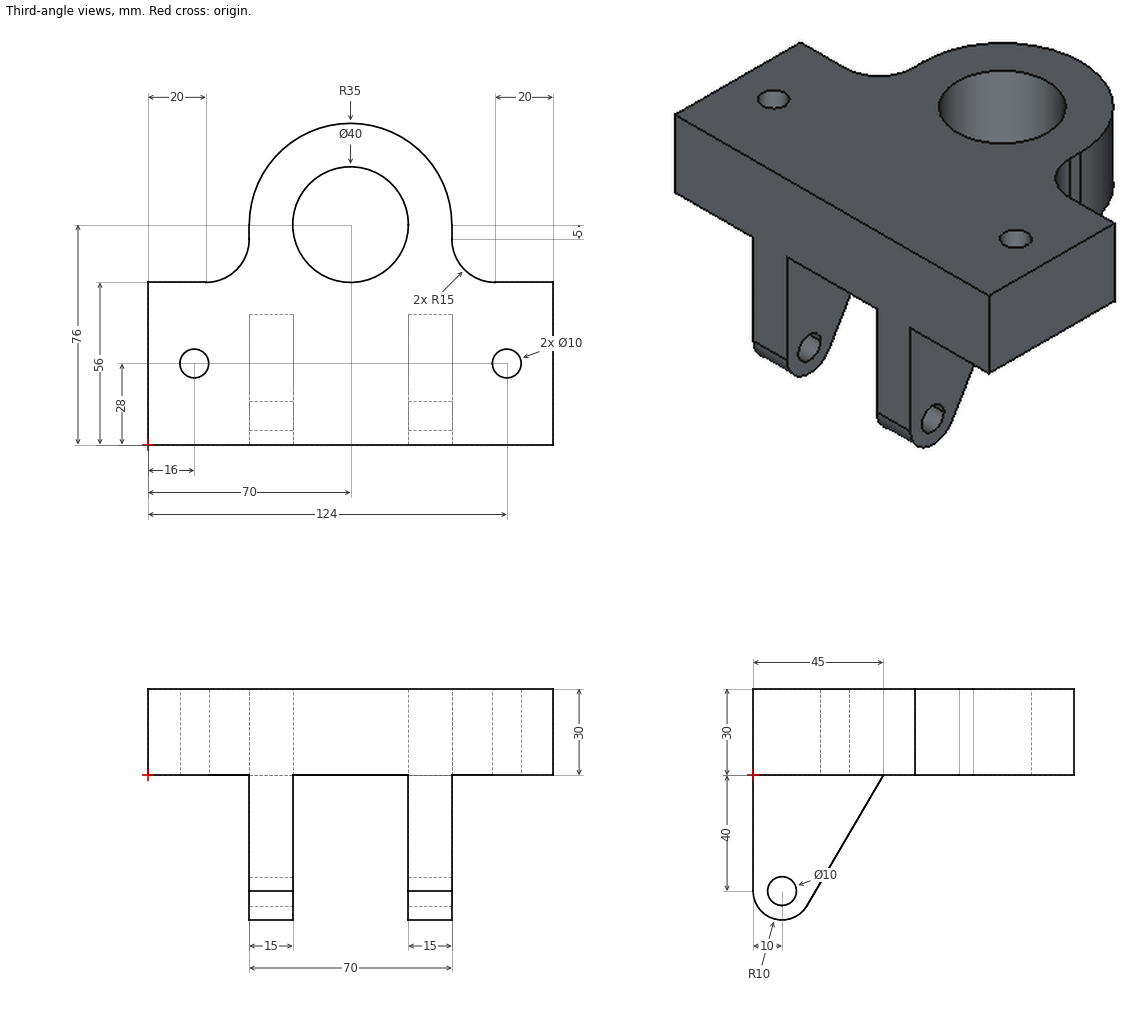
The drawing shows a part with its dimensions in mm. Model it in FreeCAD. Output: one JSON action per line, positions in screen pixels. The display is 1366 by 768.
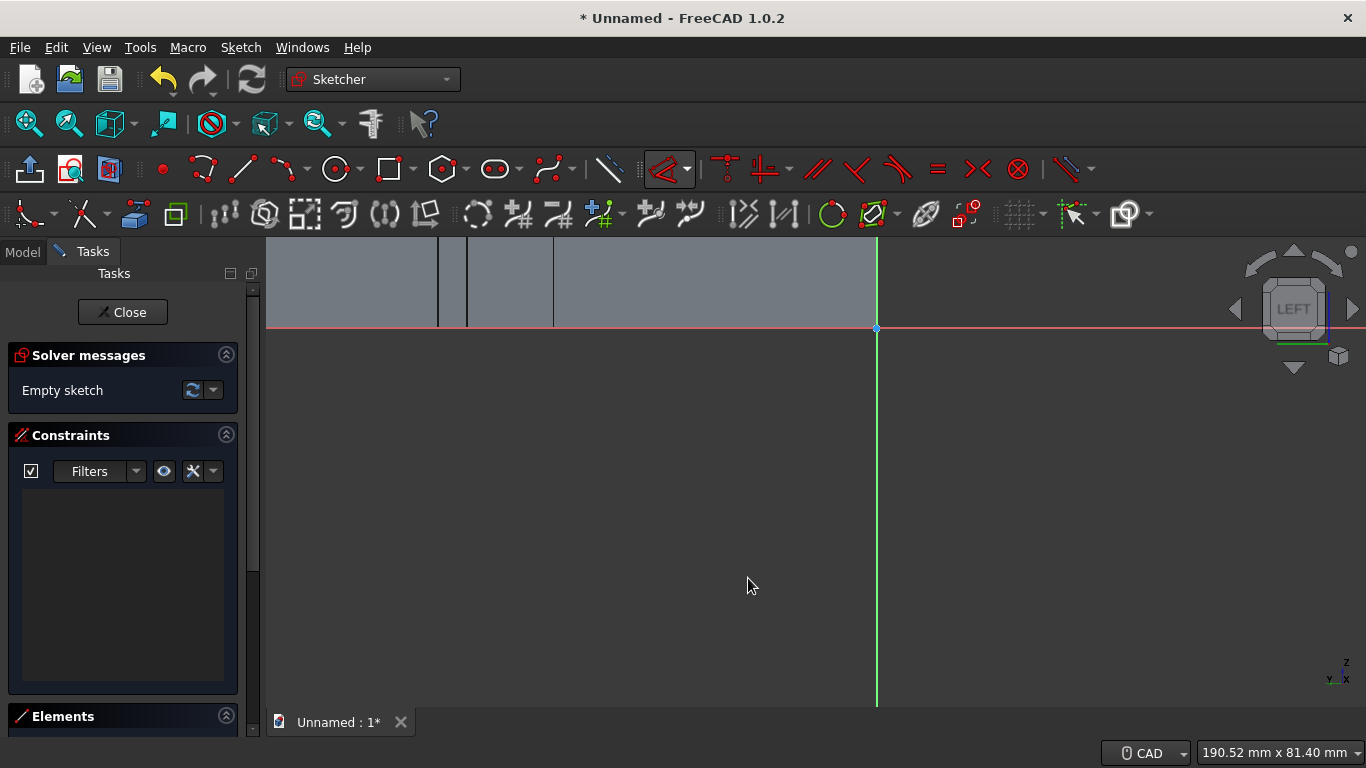
{"action": "left_click", "coordinate": [204, 170]}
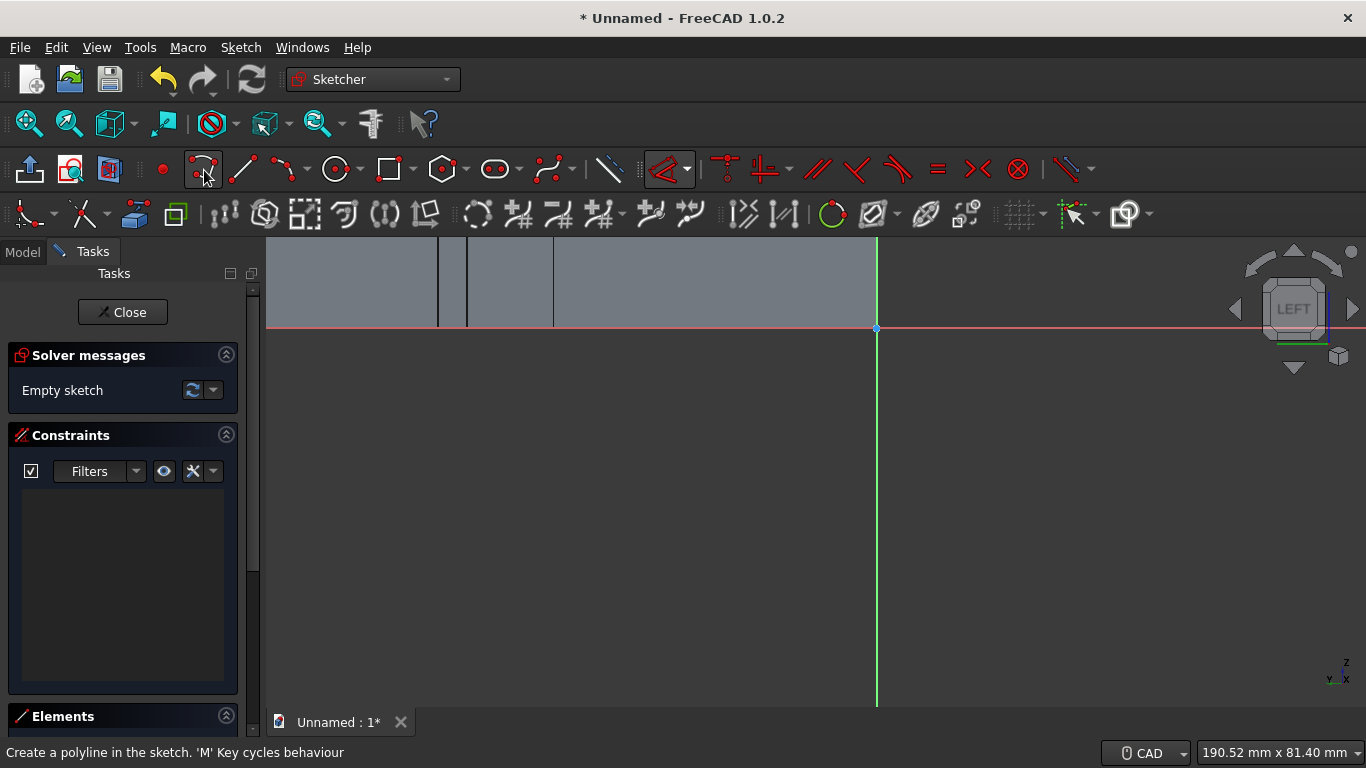
{"action": "left_click", "coordinate": [769, 588]}
{"action": "left_click", "coordinate": [617, 328]}
{"action": "left_click", "coordinate": [877, 328]}
{"action": "left_click", "coordinate": [868, 559]}
{"action": "right_click", "coordinate": [868, 559]}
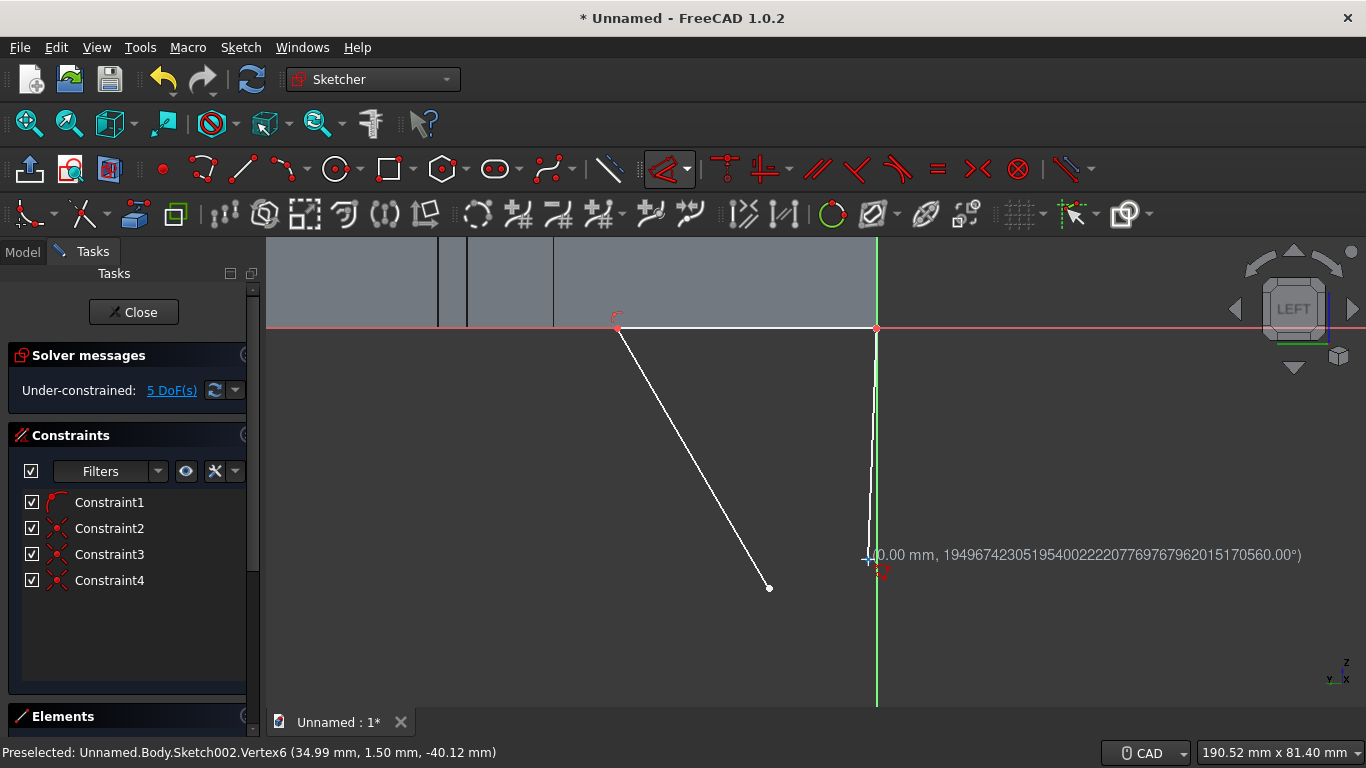
{"action": "key", "text": "g 3 a"}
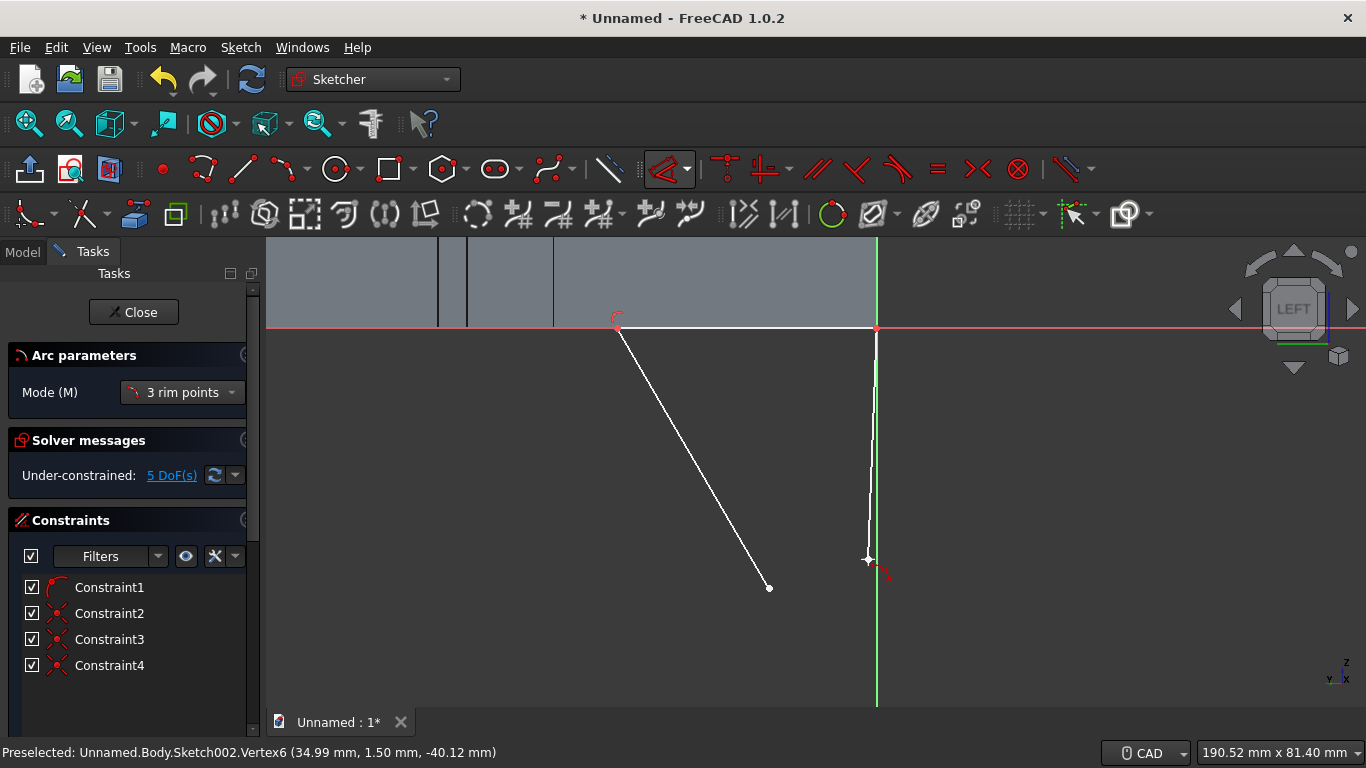
{"action": "left_click", "coordinate": [868, 560]}
{"action": "left_click", "coordinate": [769, 589]}
{"action": "left_click", "coordinate": [834, 615]}
{"action": "key", "text": "Escape"}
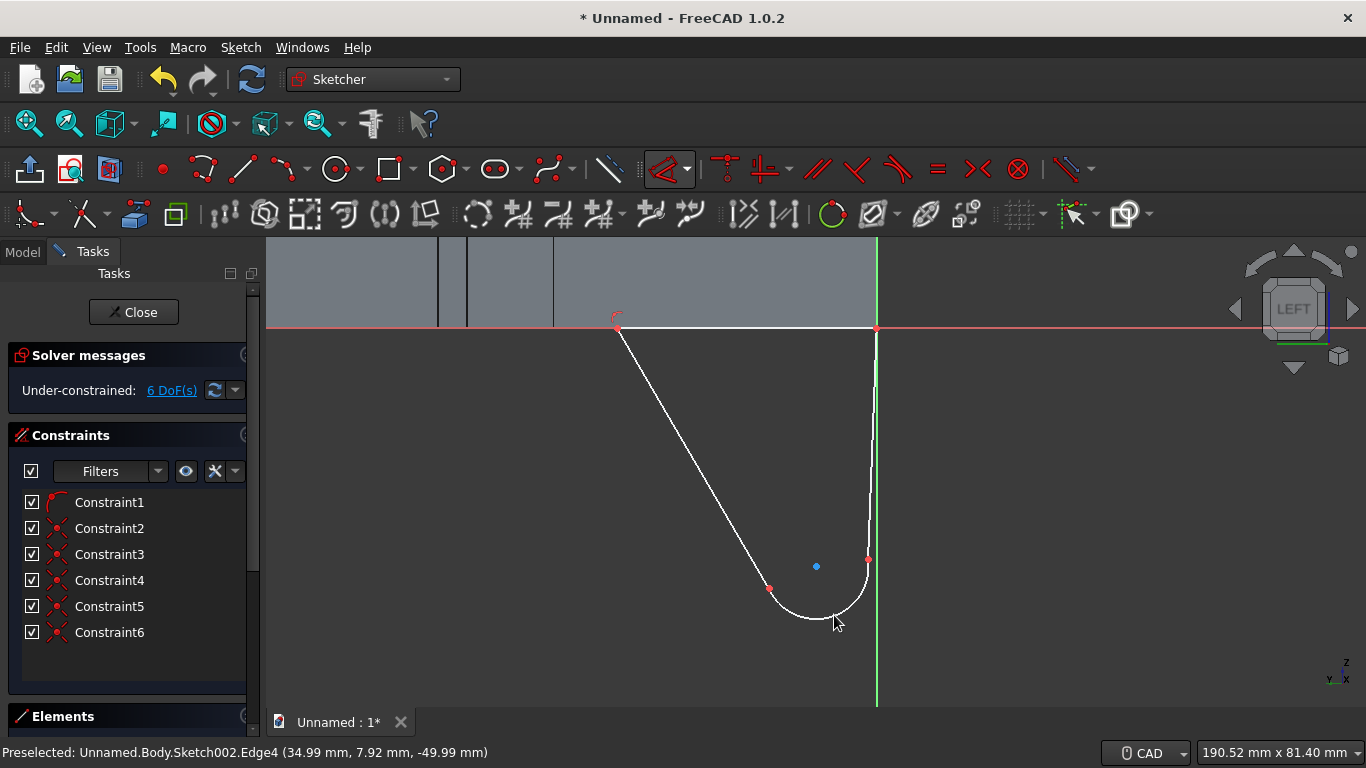
{"action": "left_click", "coordinate": [723, 511]}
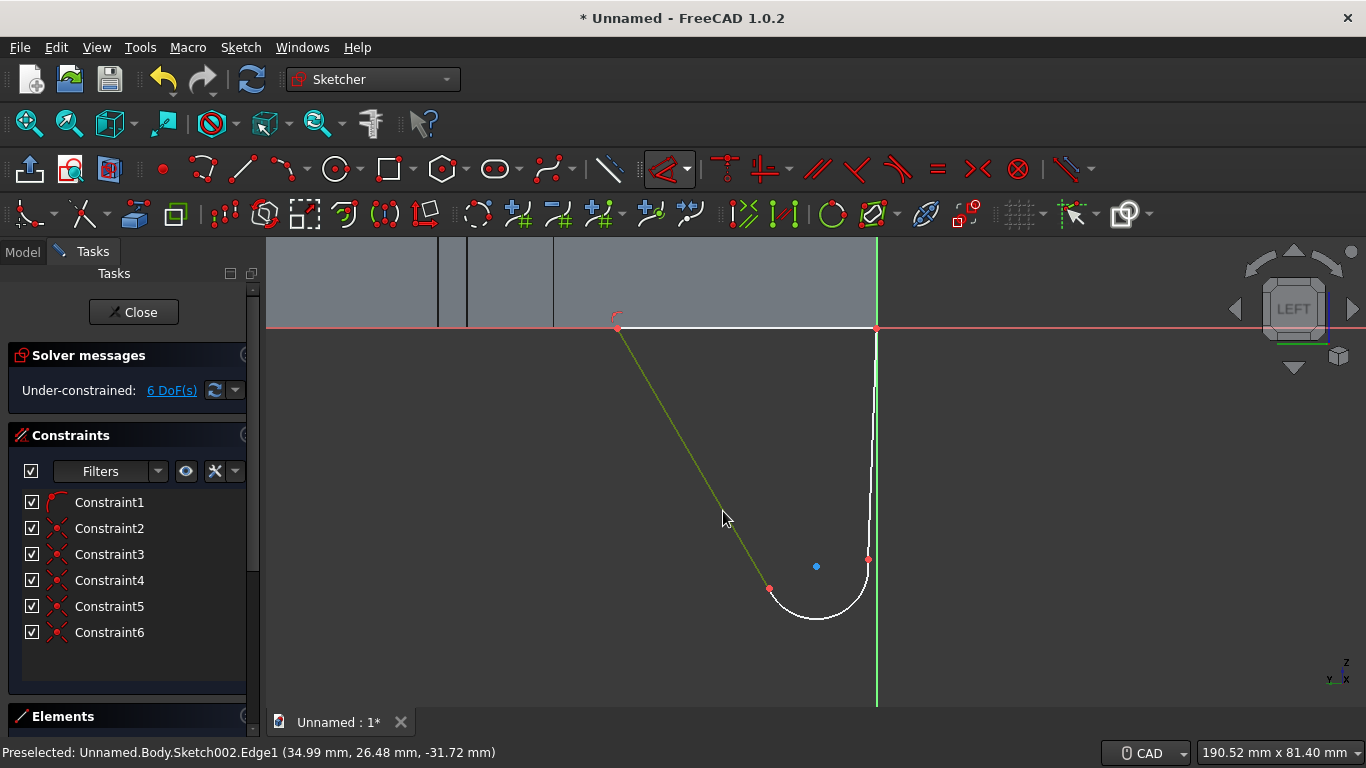
{"action": "left_click", "coordinate": [802, 617]}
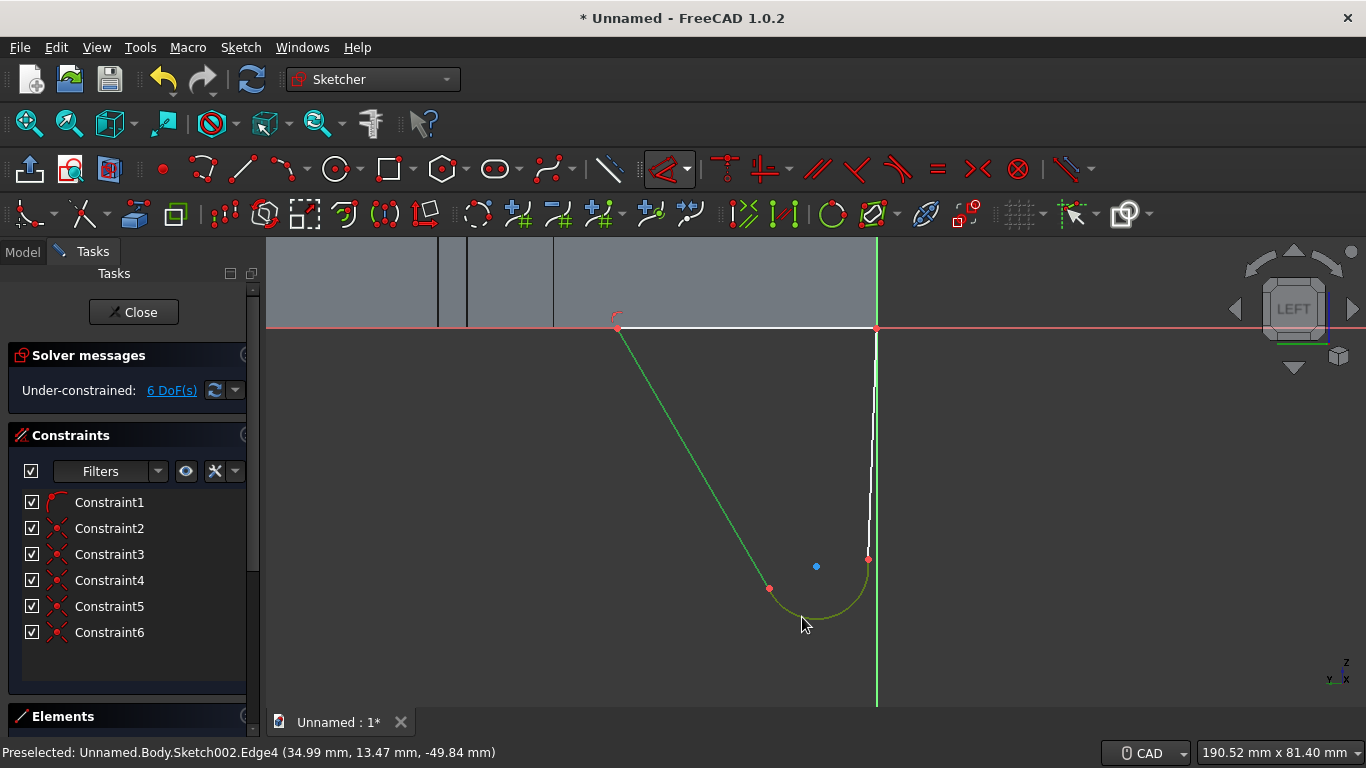
{"action": "left_click", "coordinate": [898, 170]}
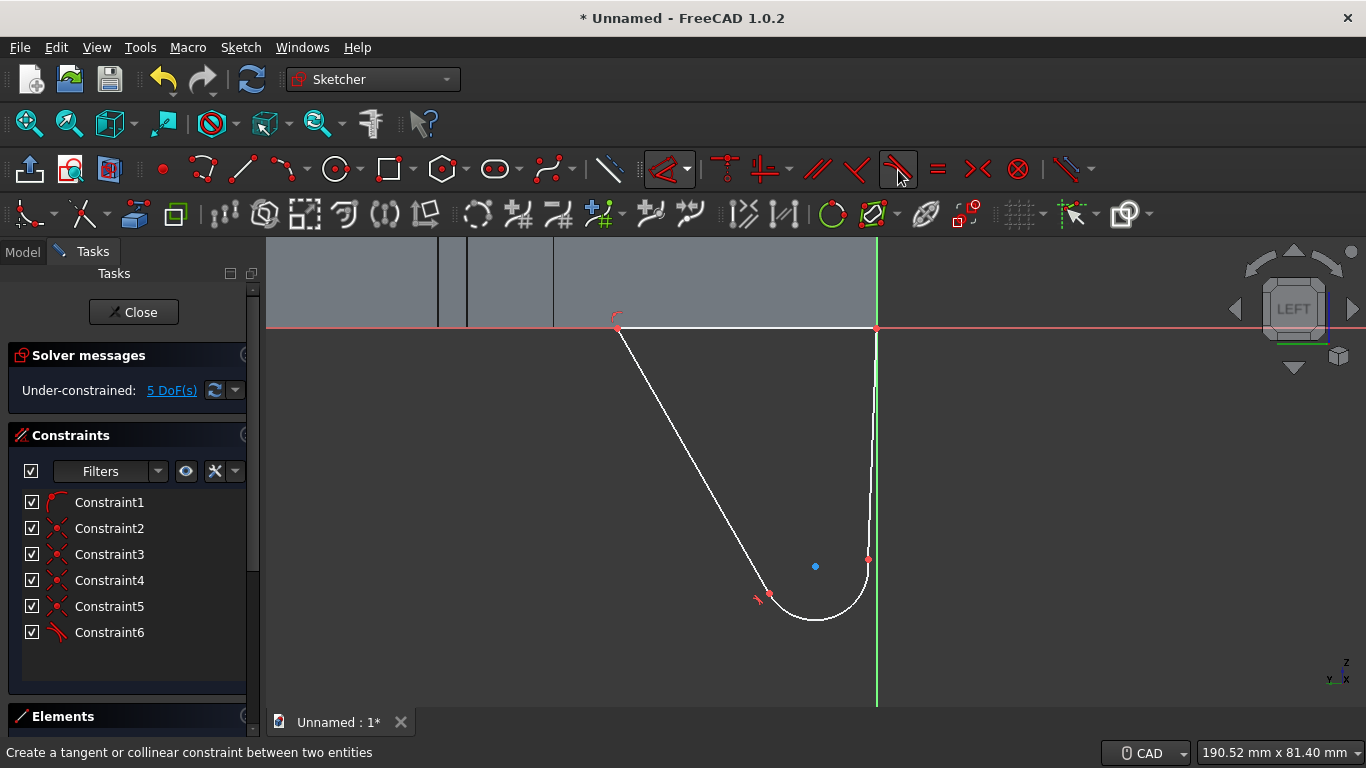
{"action": "left_click", "coordinate": [874, 398]}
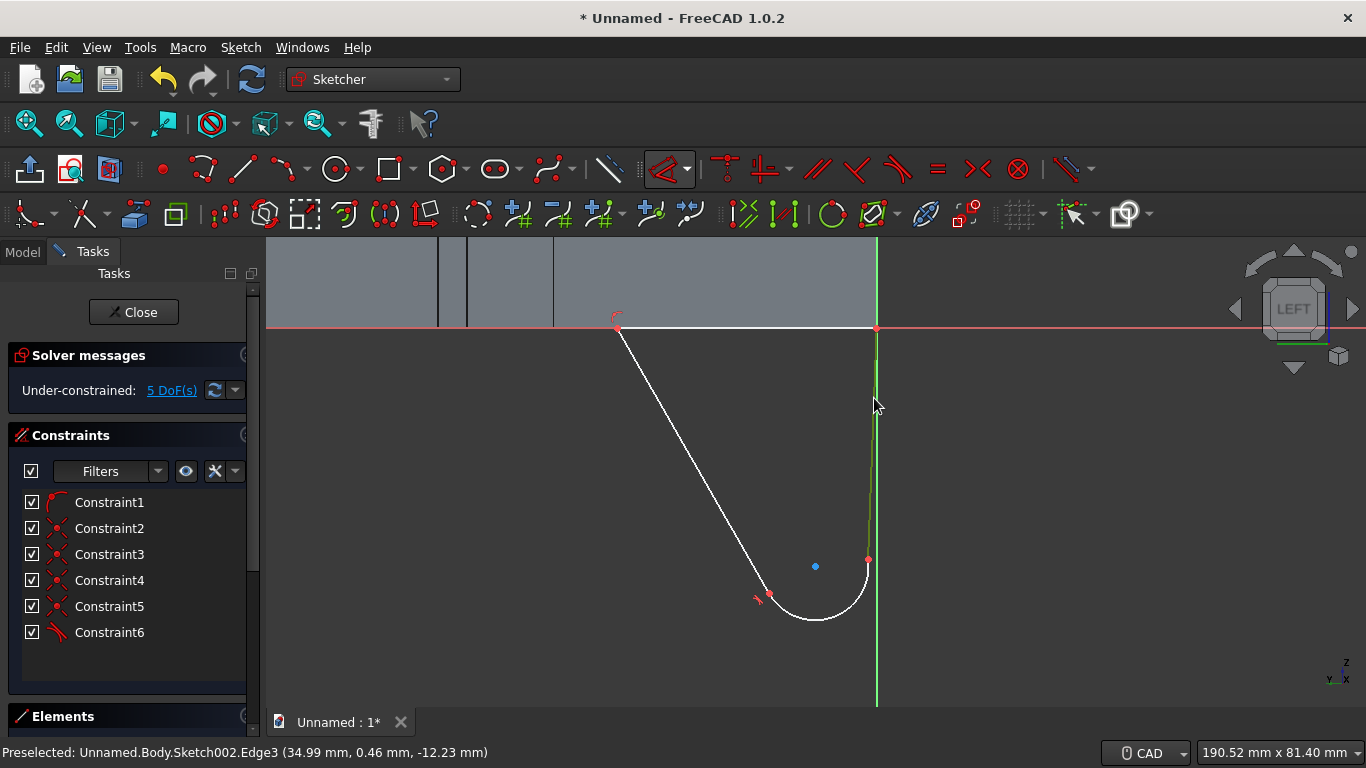
{"action": "left_click", "coordinate": [803, 619]}